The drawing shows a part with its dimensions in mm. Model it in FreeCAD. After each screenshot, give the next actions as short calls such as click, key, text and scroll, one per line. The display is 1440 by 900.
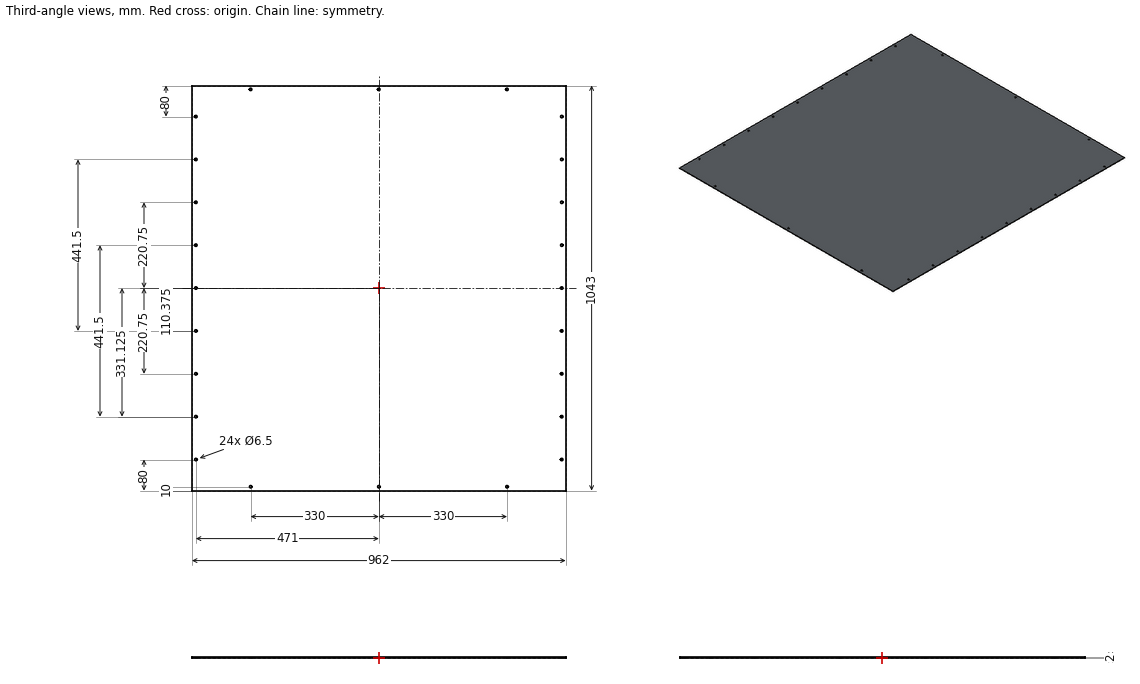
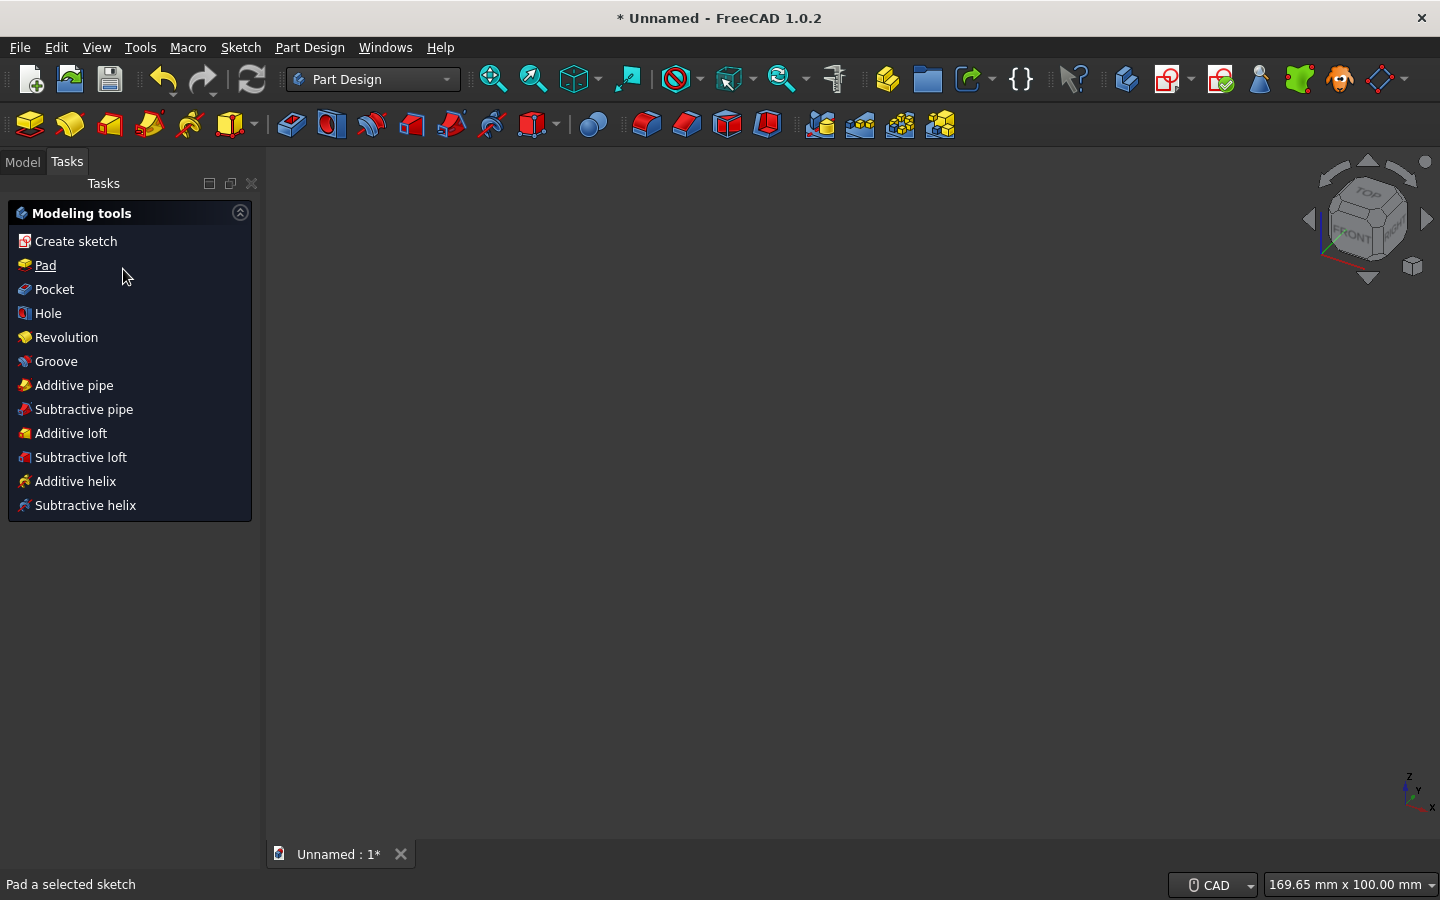
click(30, 124)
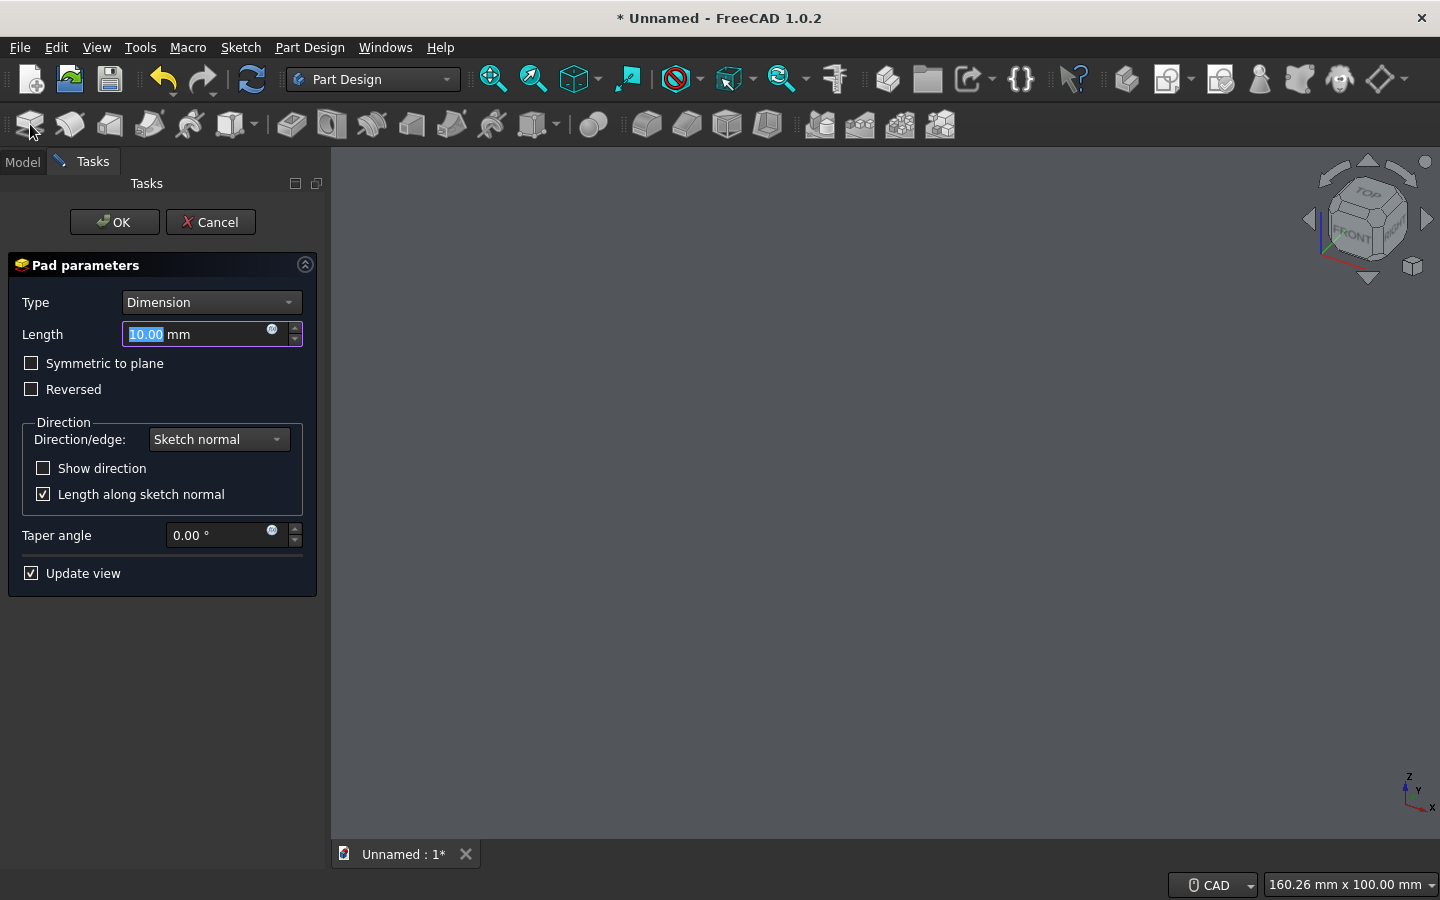
text(2)
key(Tab)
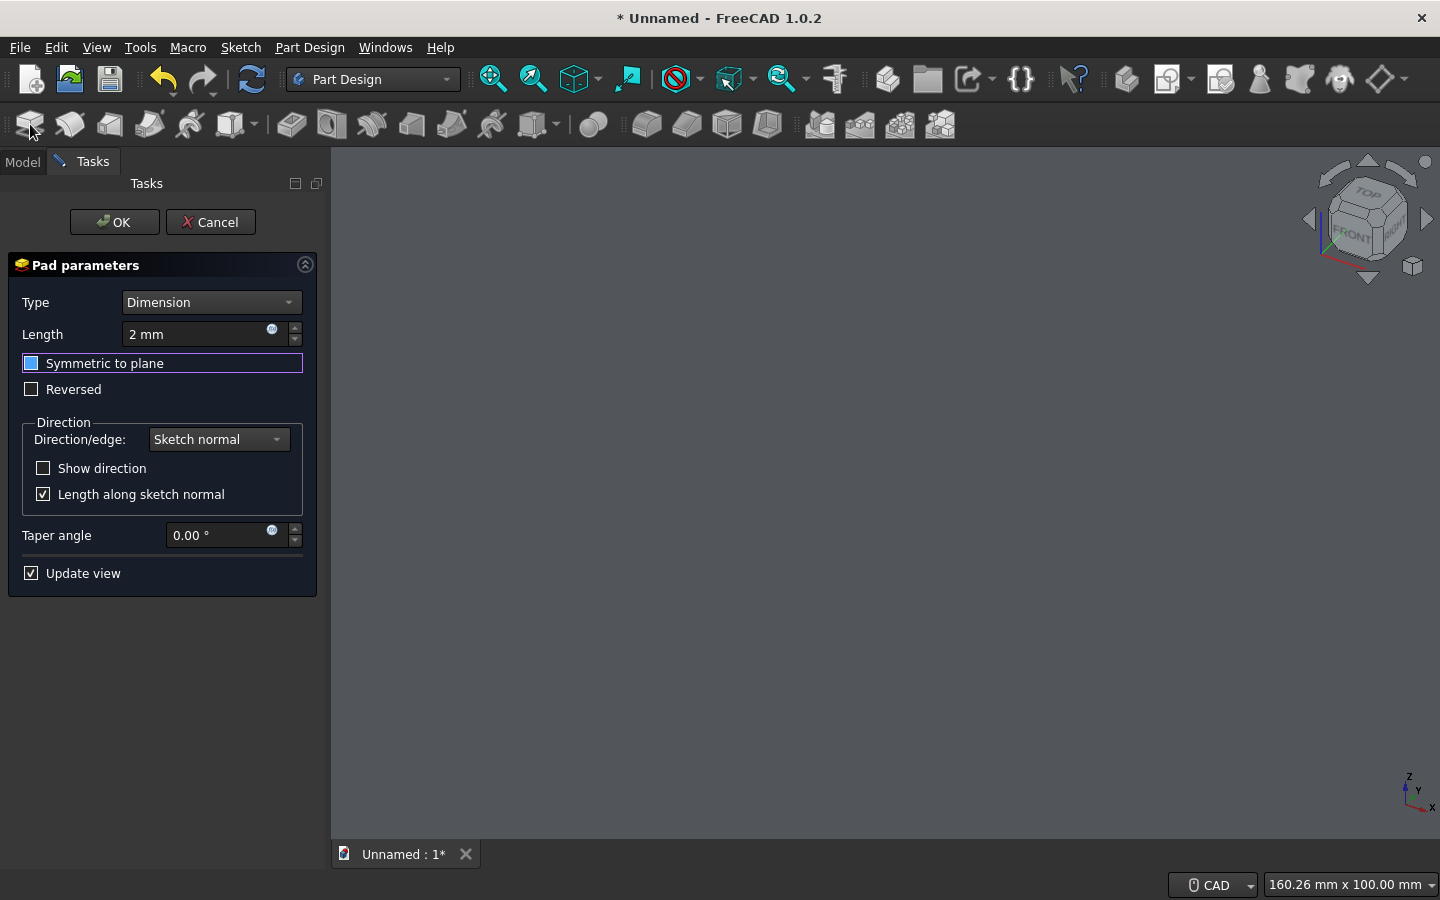
click(115, 222)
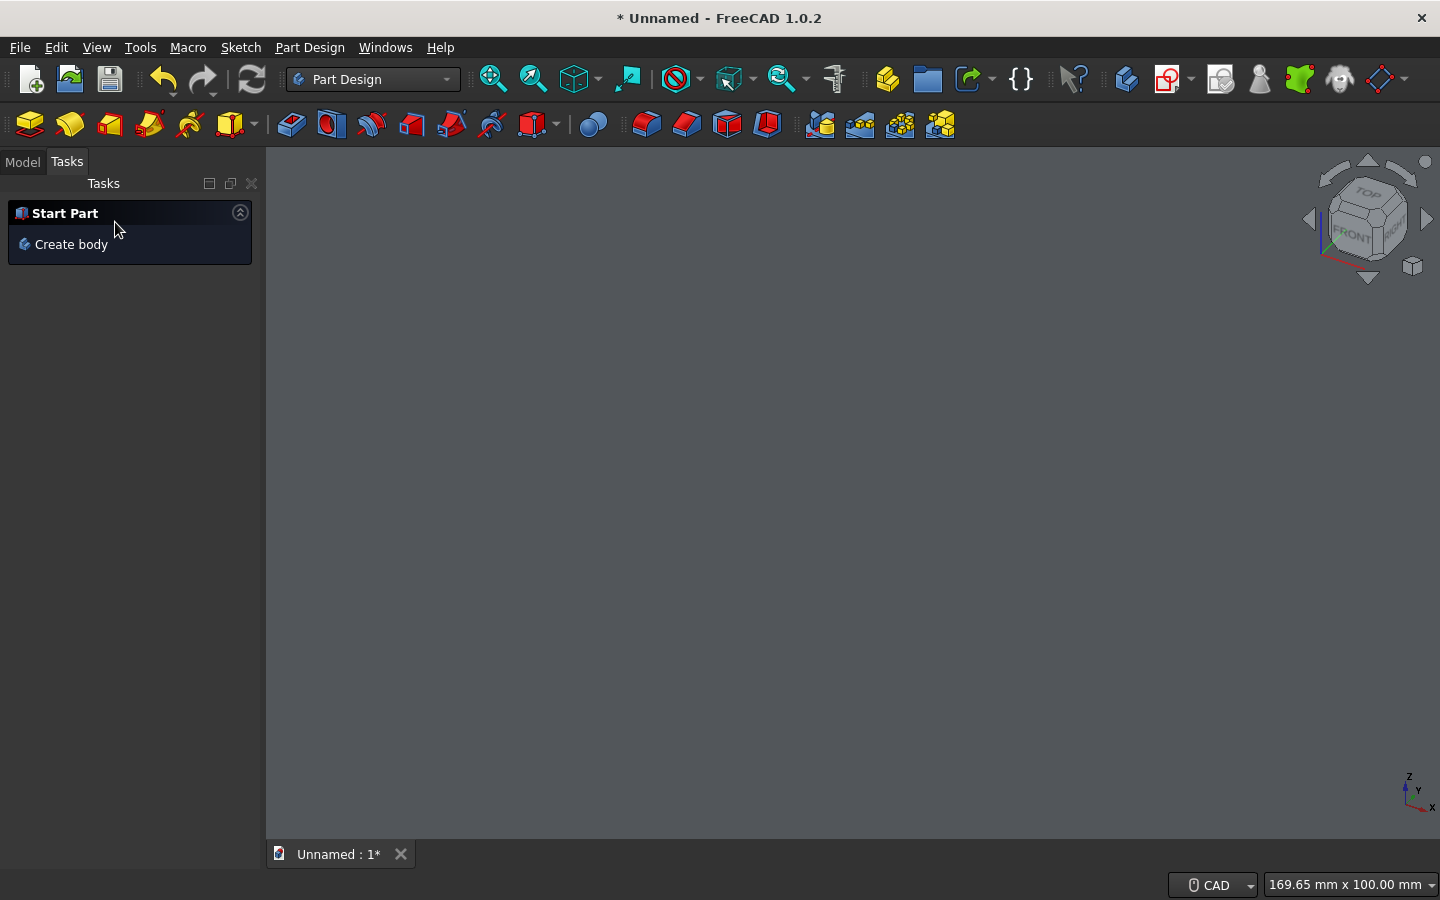
key(0)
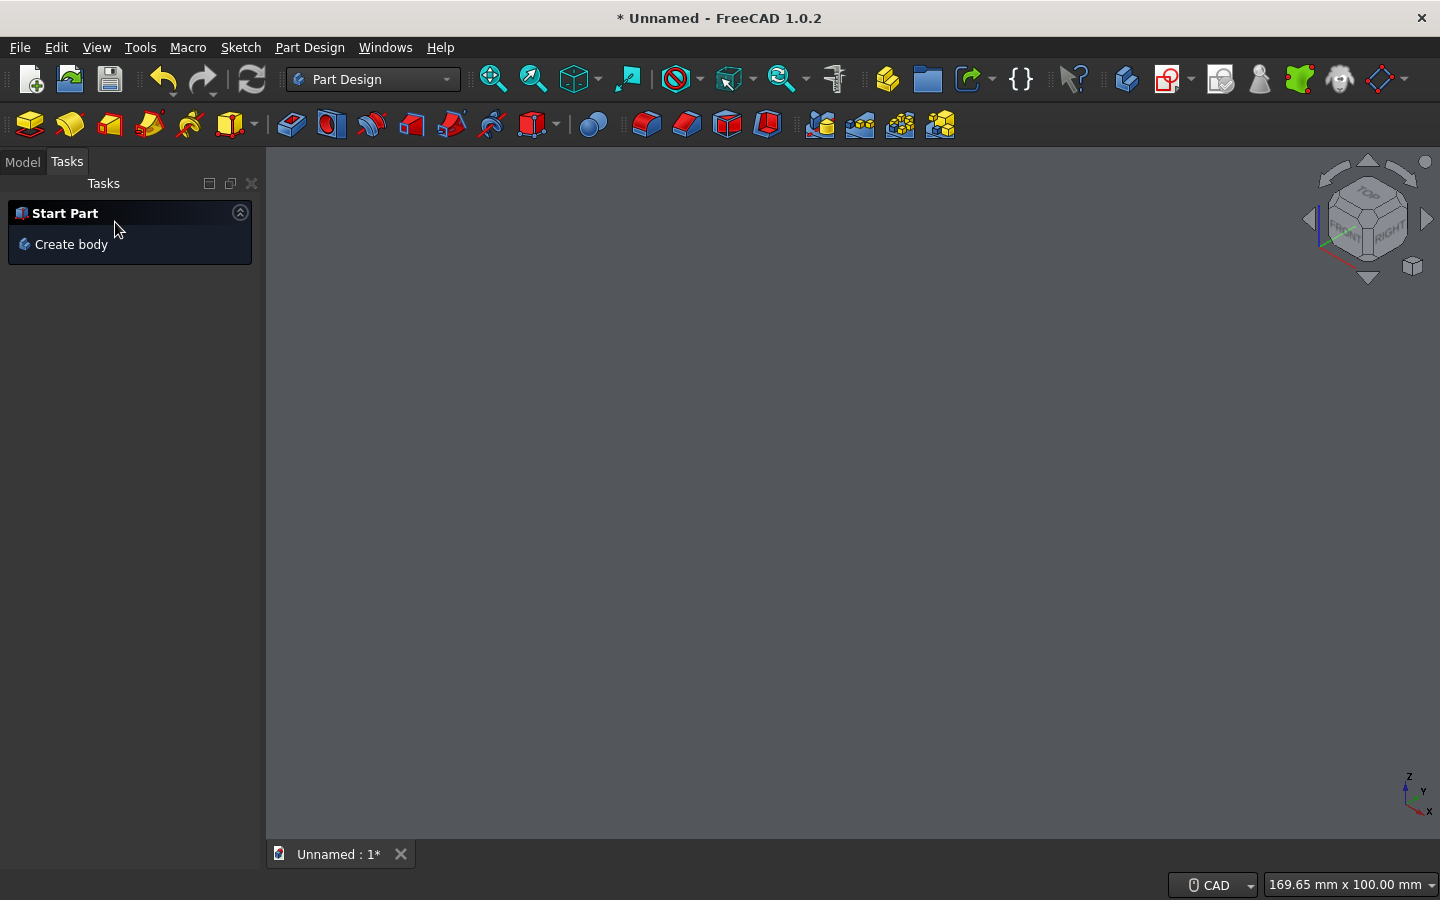
click(494, 80)